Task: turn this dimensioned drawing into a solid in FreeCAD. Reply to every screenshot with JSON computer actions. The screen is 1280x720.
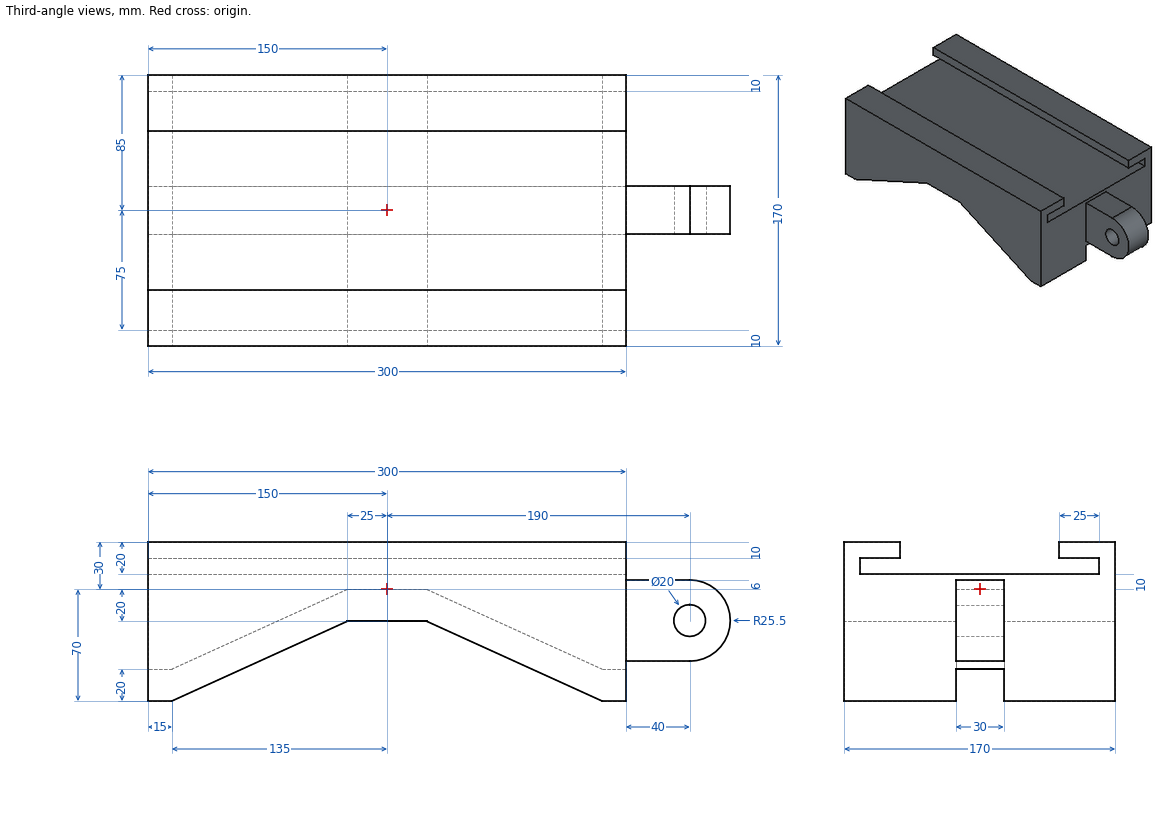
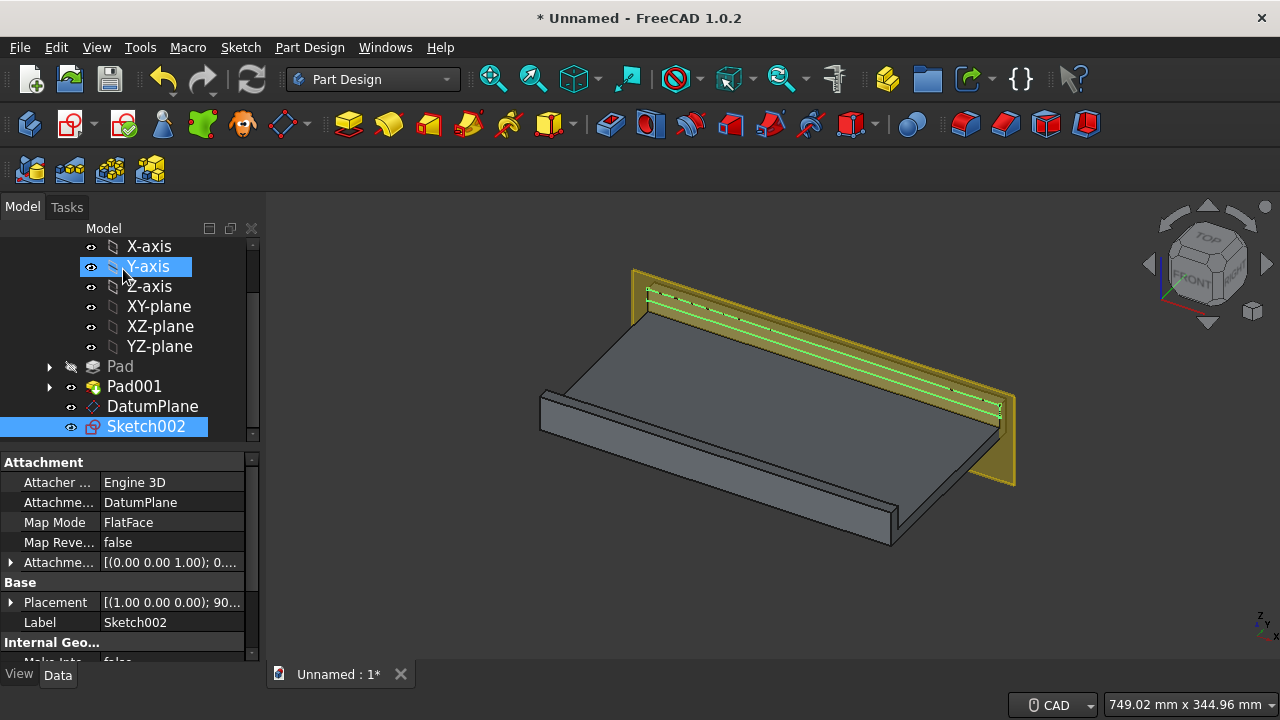
{"action": "left_click", "coordinate": [350, 124]}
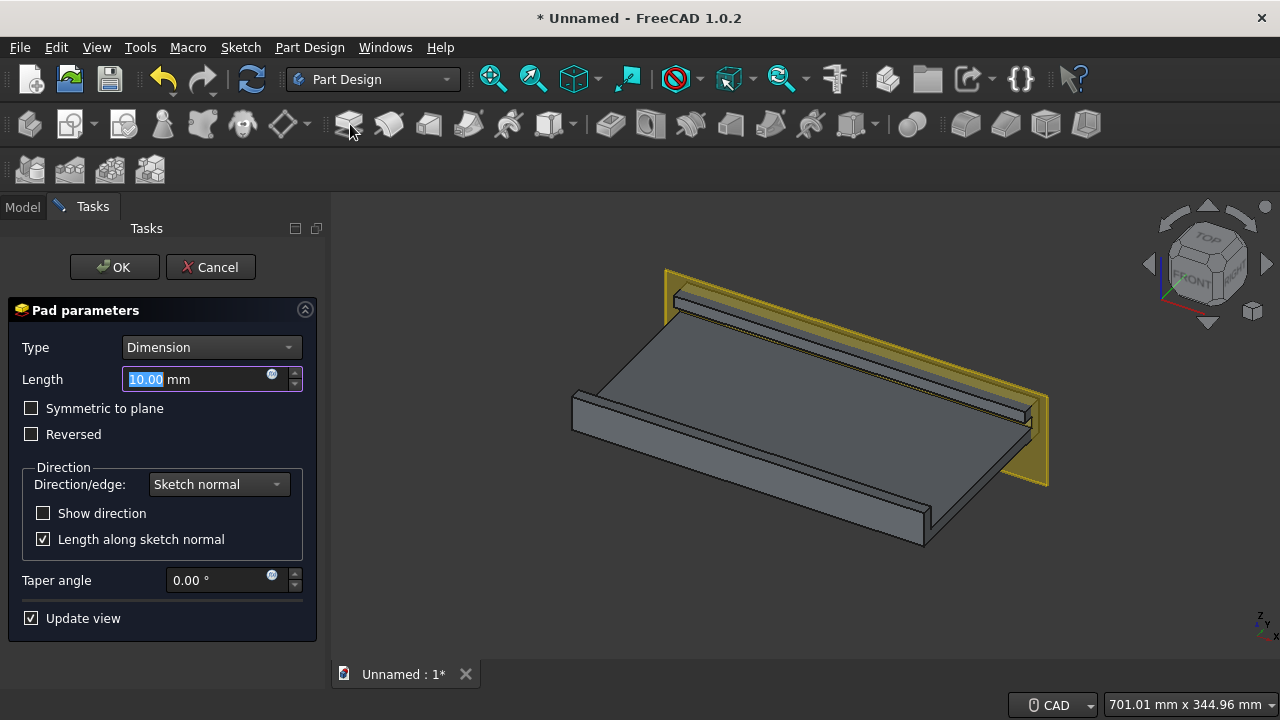
{"action": "type", "text": "25"}
{"action": "key", "text": "Tab"}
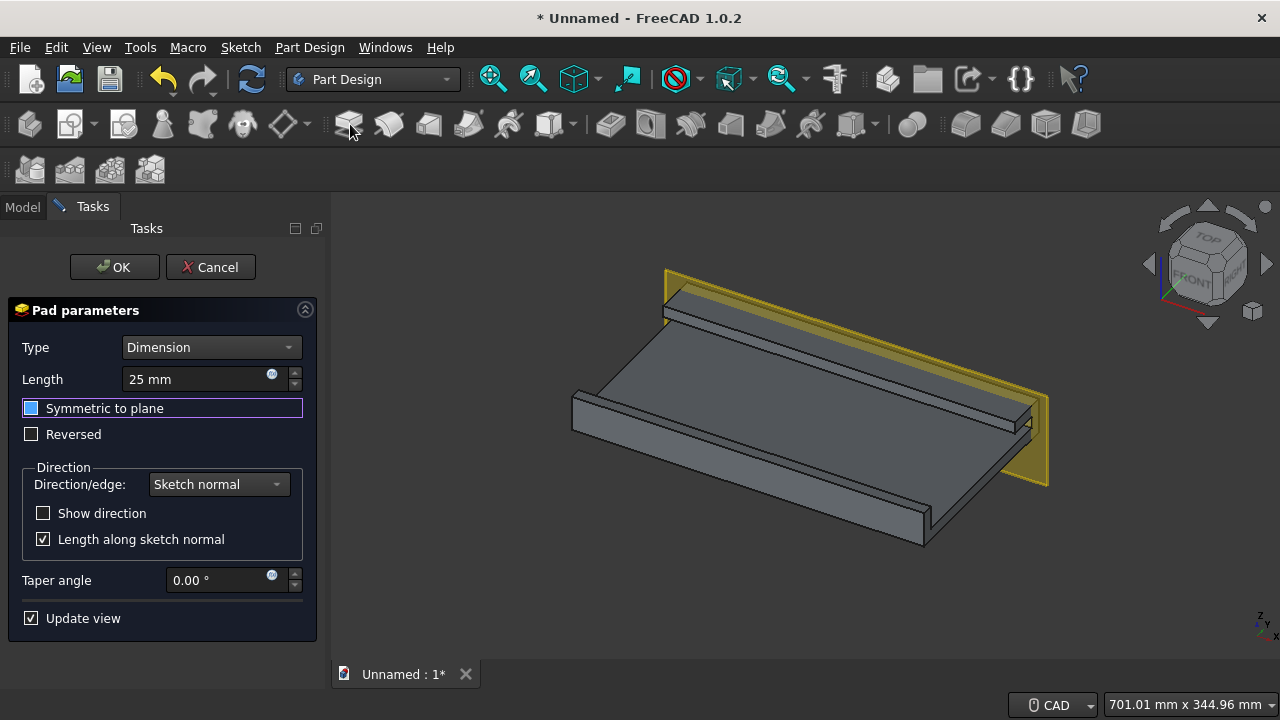
{"action": "left_click", "coordinate": [115, 267]}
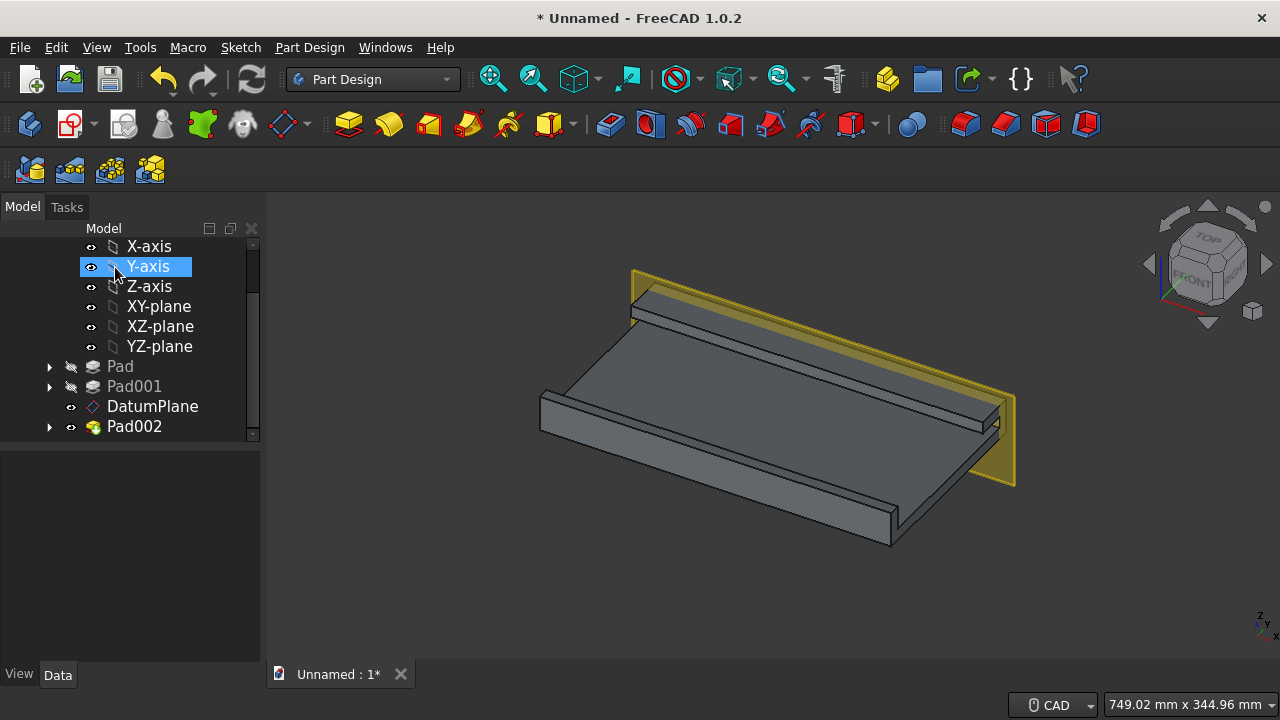
{"action": "left_click", "coordinate": [116, 407]}
{"action": "key", "text": "space"}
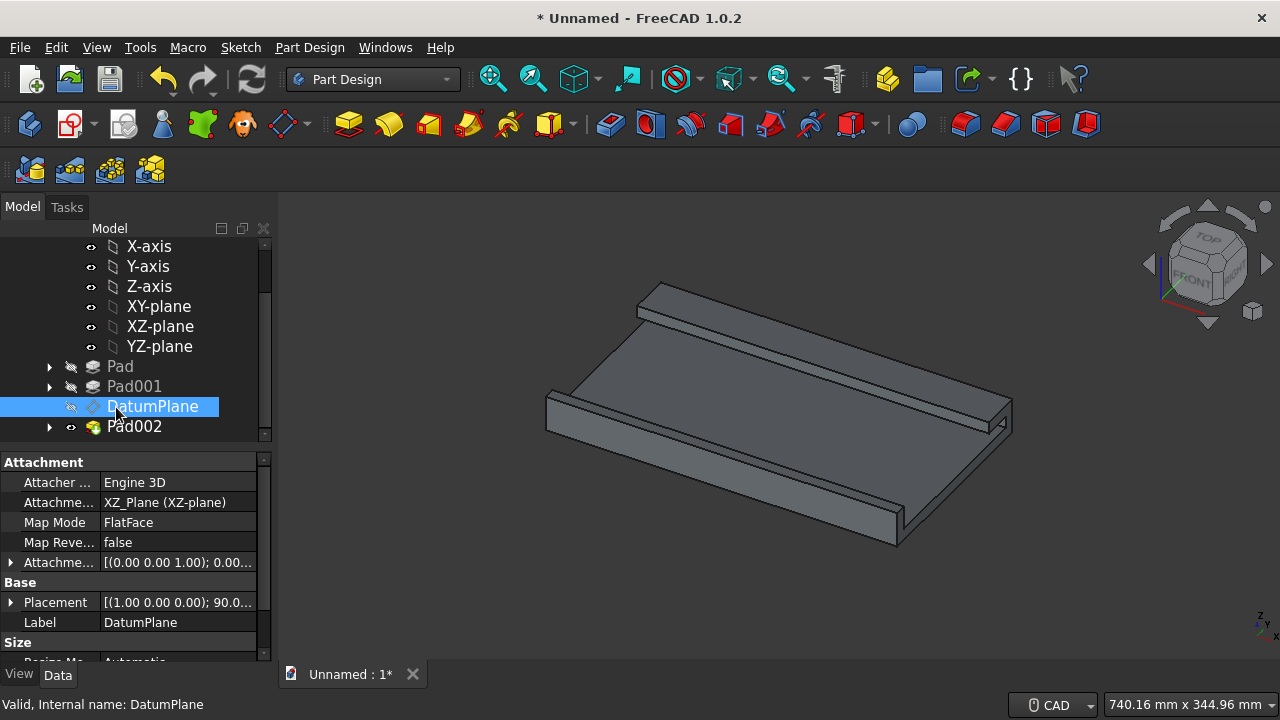
{"action": "left_click", "coordinate": [116, 427]}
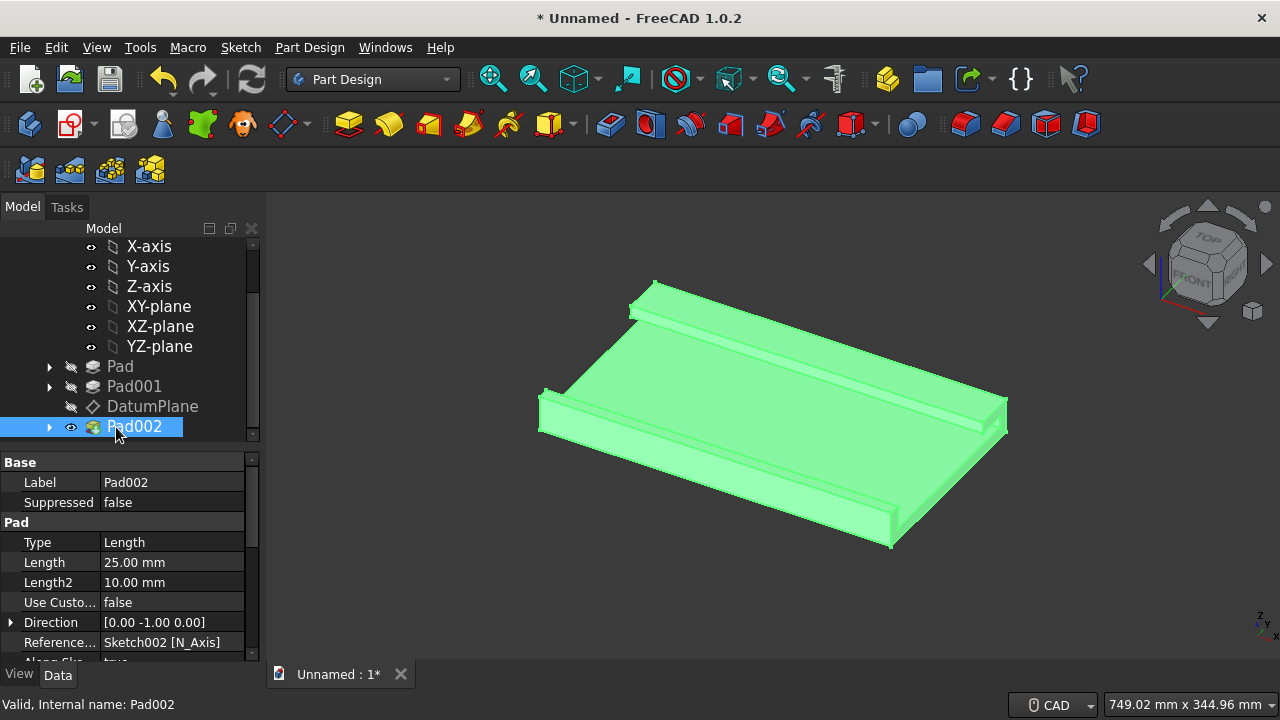
{"action": "left_click", "coordinate": [30, 170]}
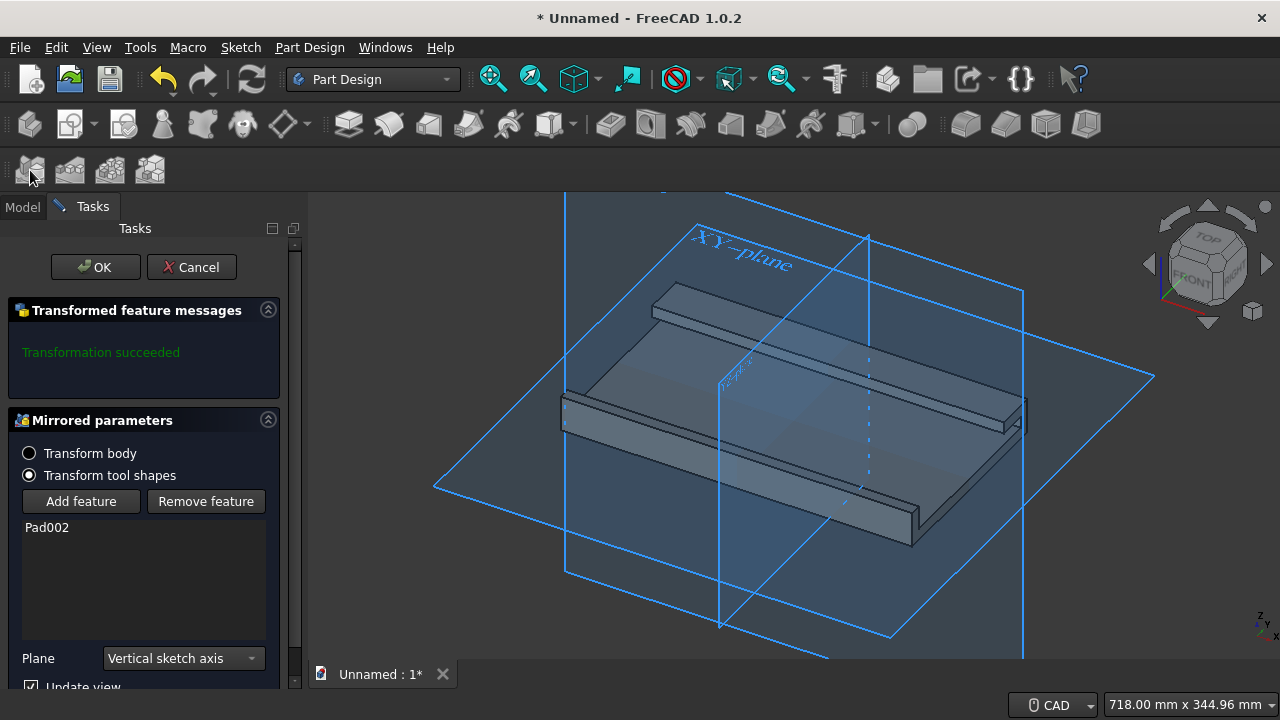
{"action": "left_click", "coordinate": [184, 658]}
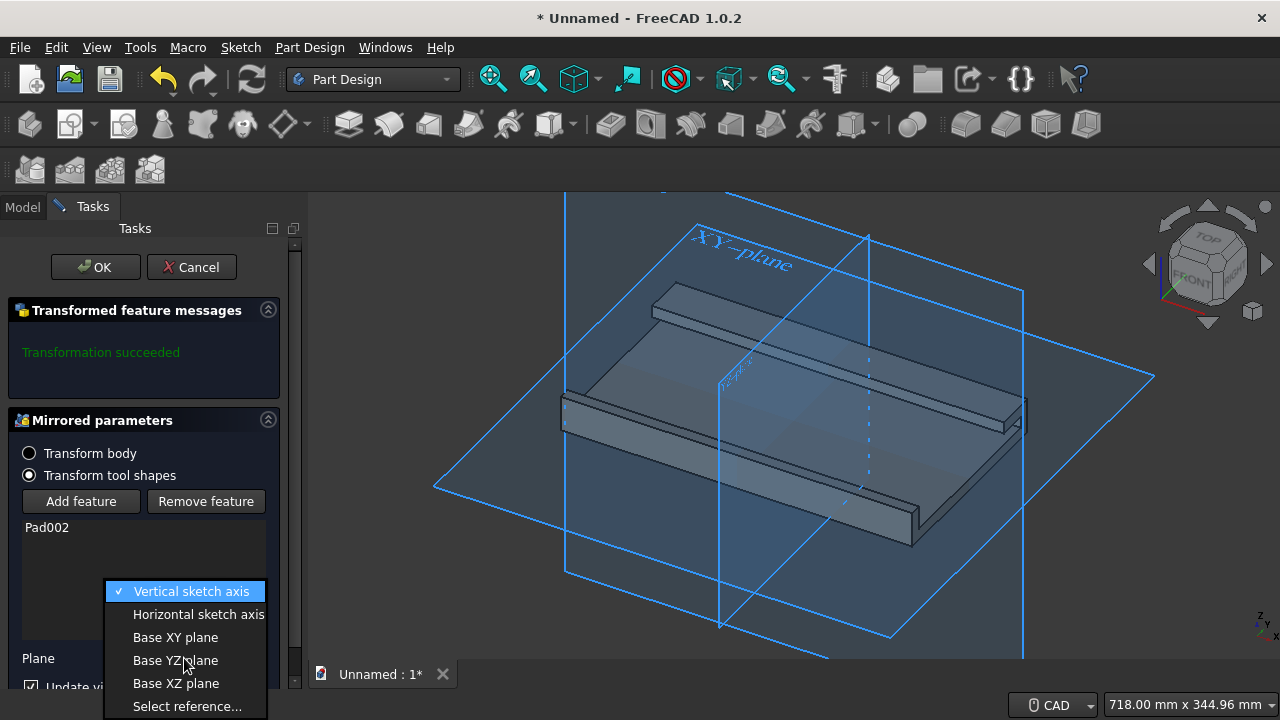
{"action": "left_click", "coordinate": [184, 684]}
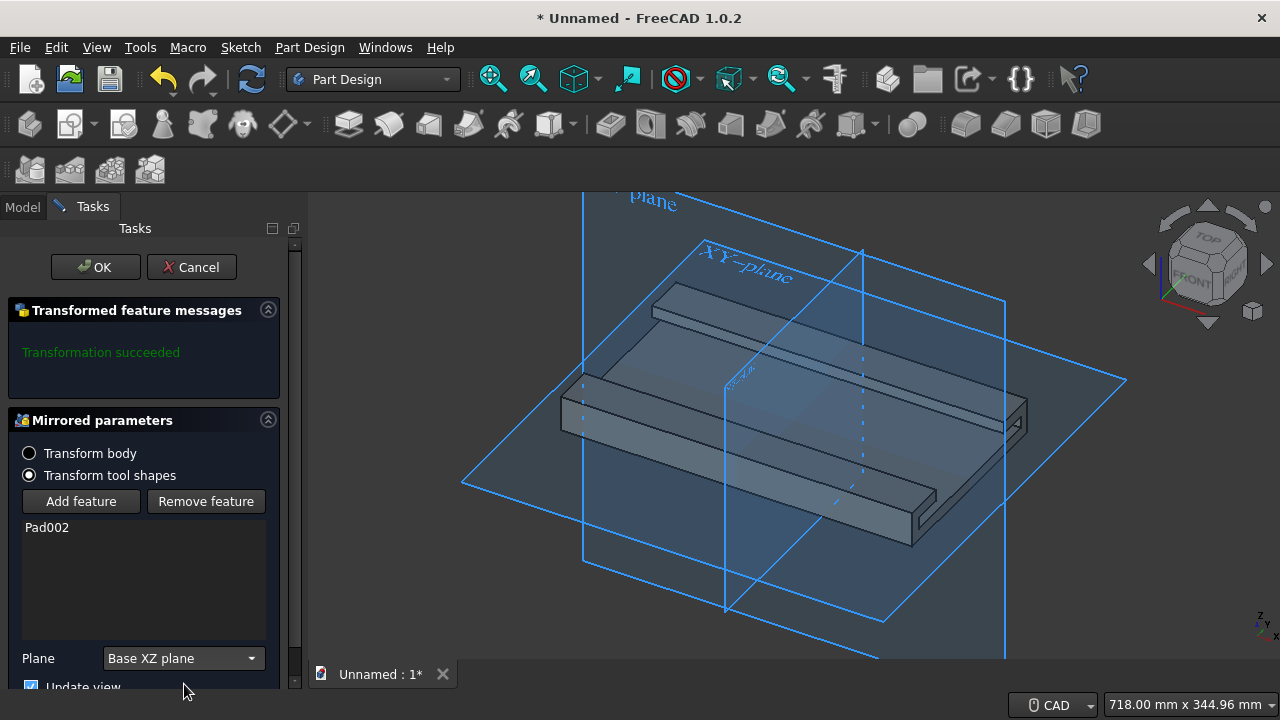
{"action": "left_click", "coordinate": [96, 267]}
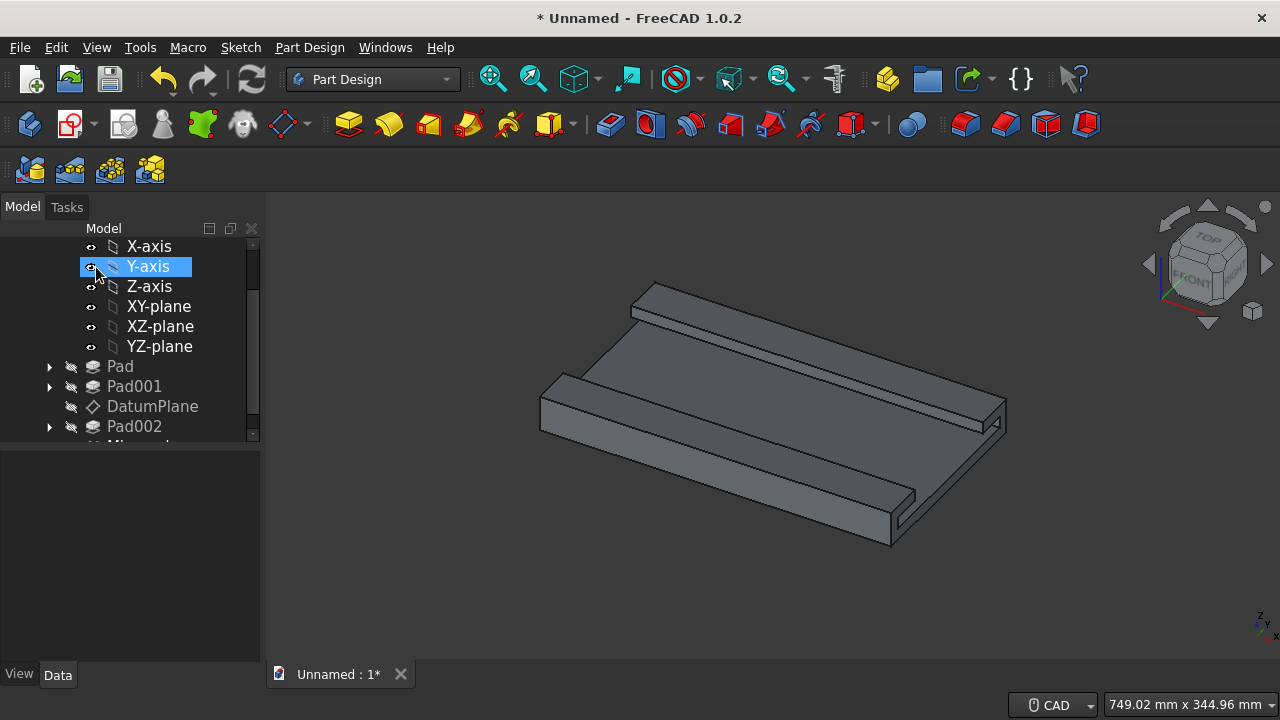
{"action": "left_click", "coordinate": [70, 124]}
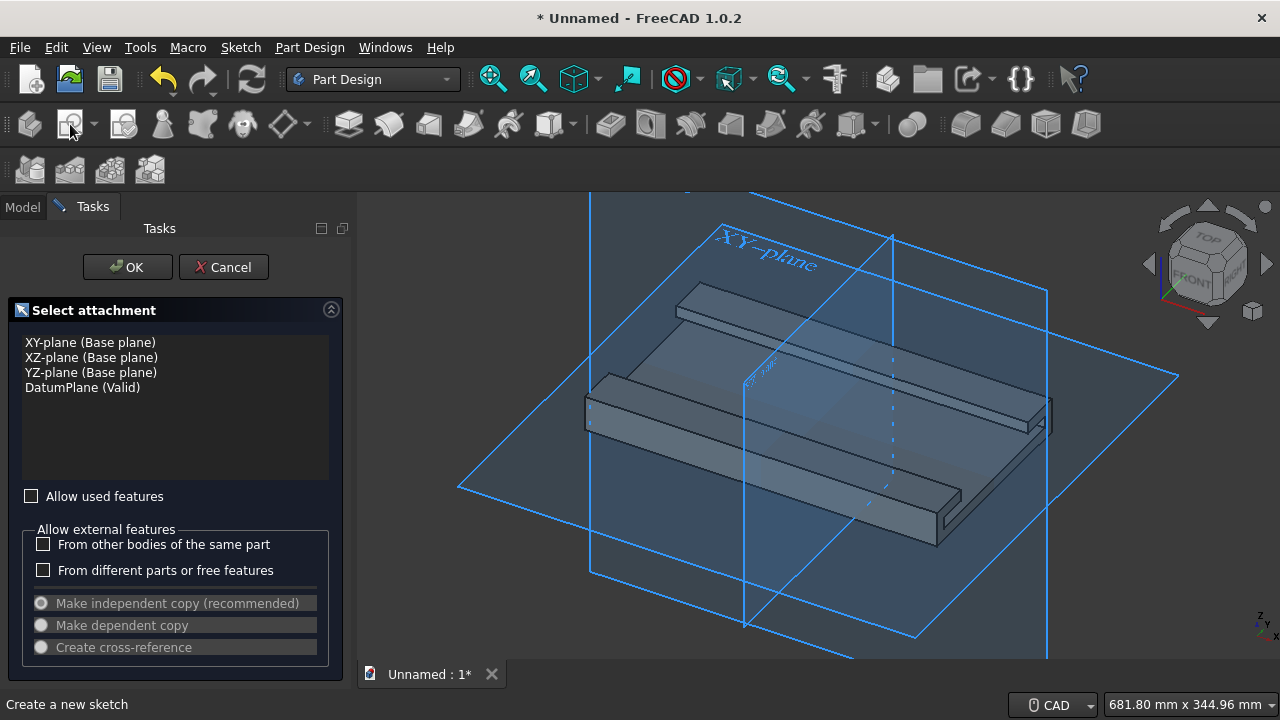
{"action": "left_click", "coordinate": [82, 358]}